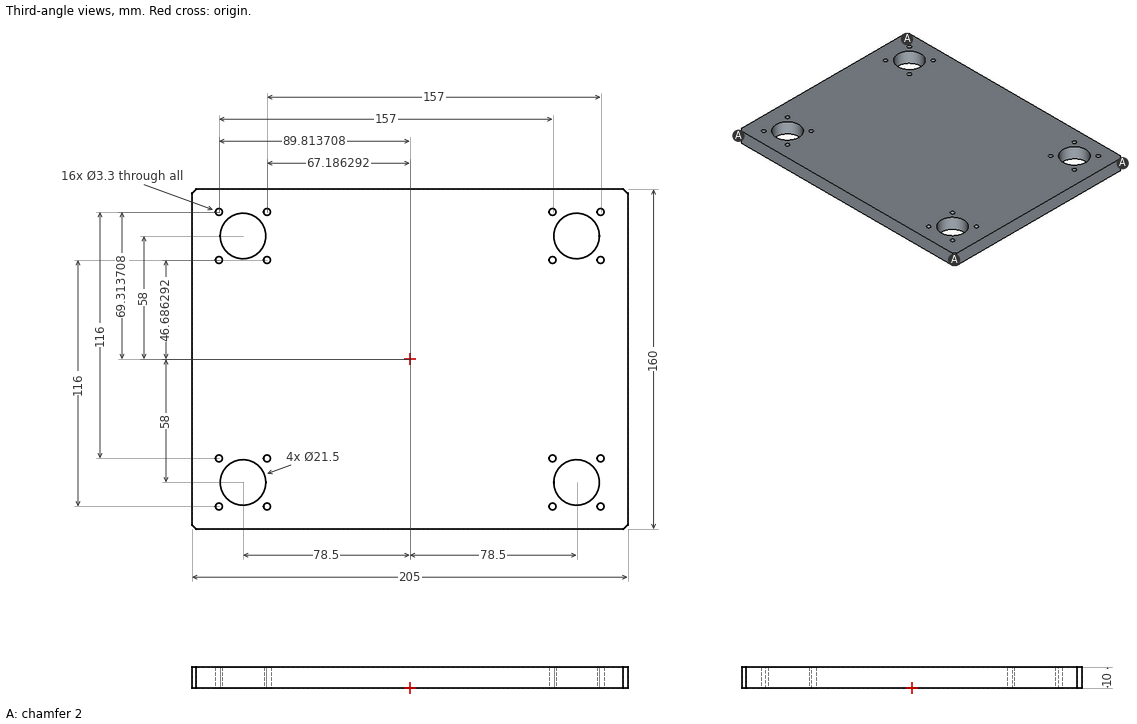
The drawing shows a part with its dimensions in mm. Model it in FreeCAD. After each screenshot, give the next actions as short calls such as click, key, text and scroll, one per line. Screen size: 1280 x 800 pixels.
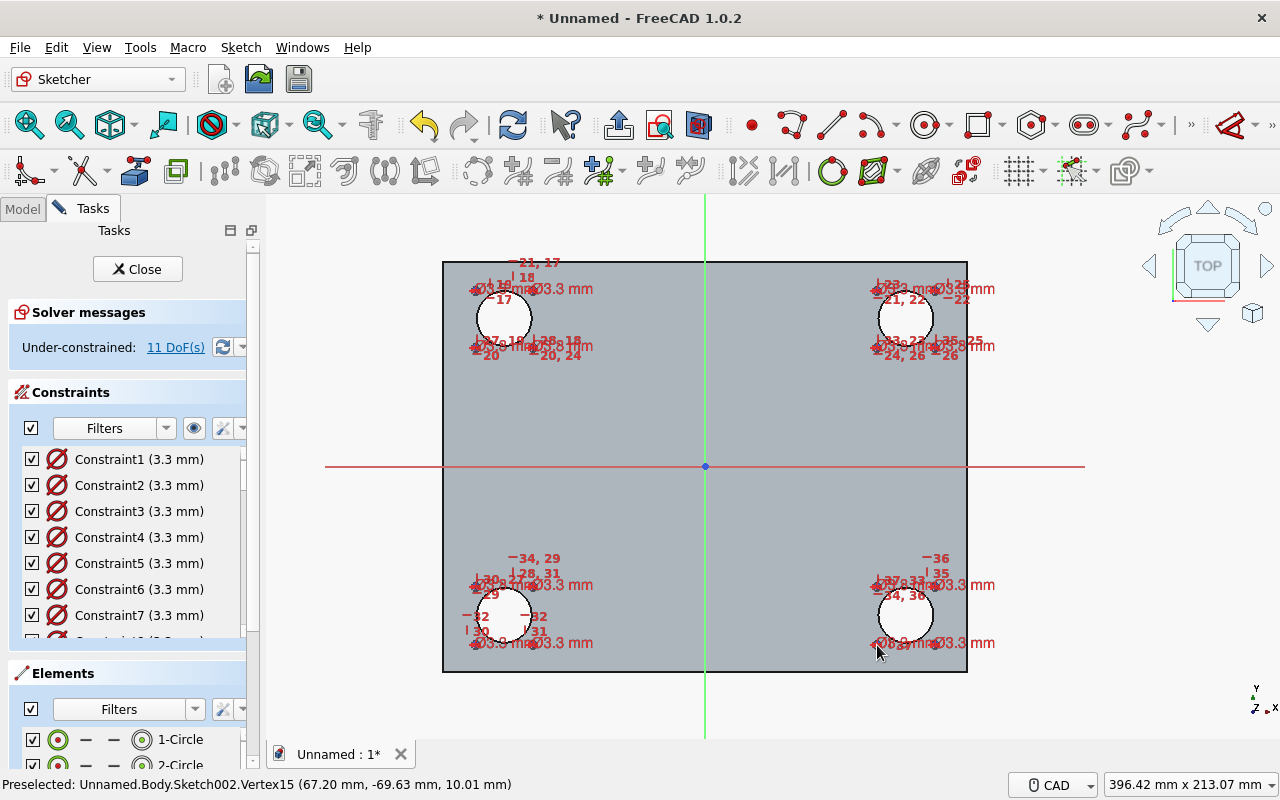
click(533, 645)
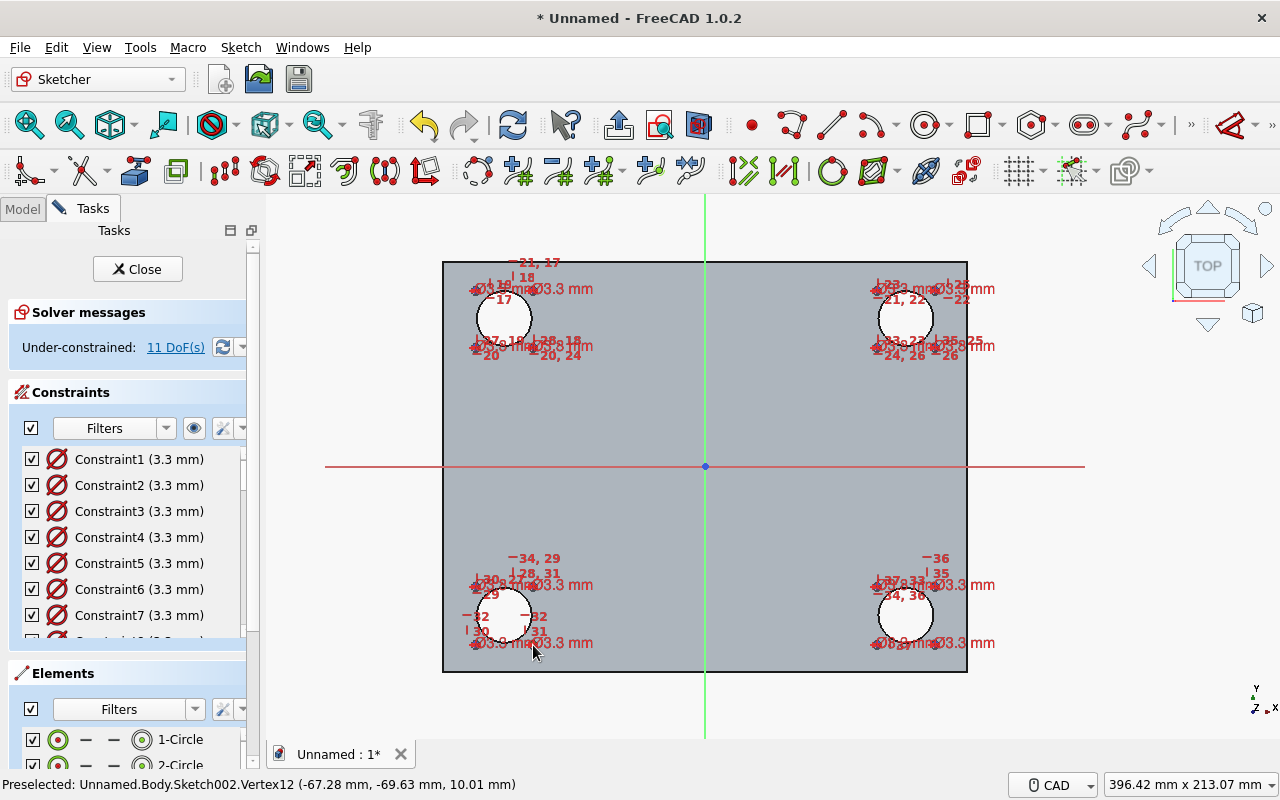
click(877, 645)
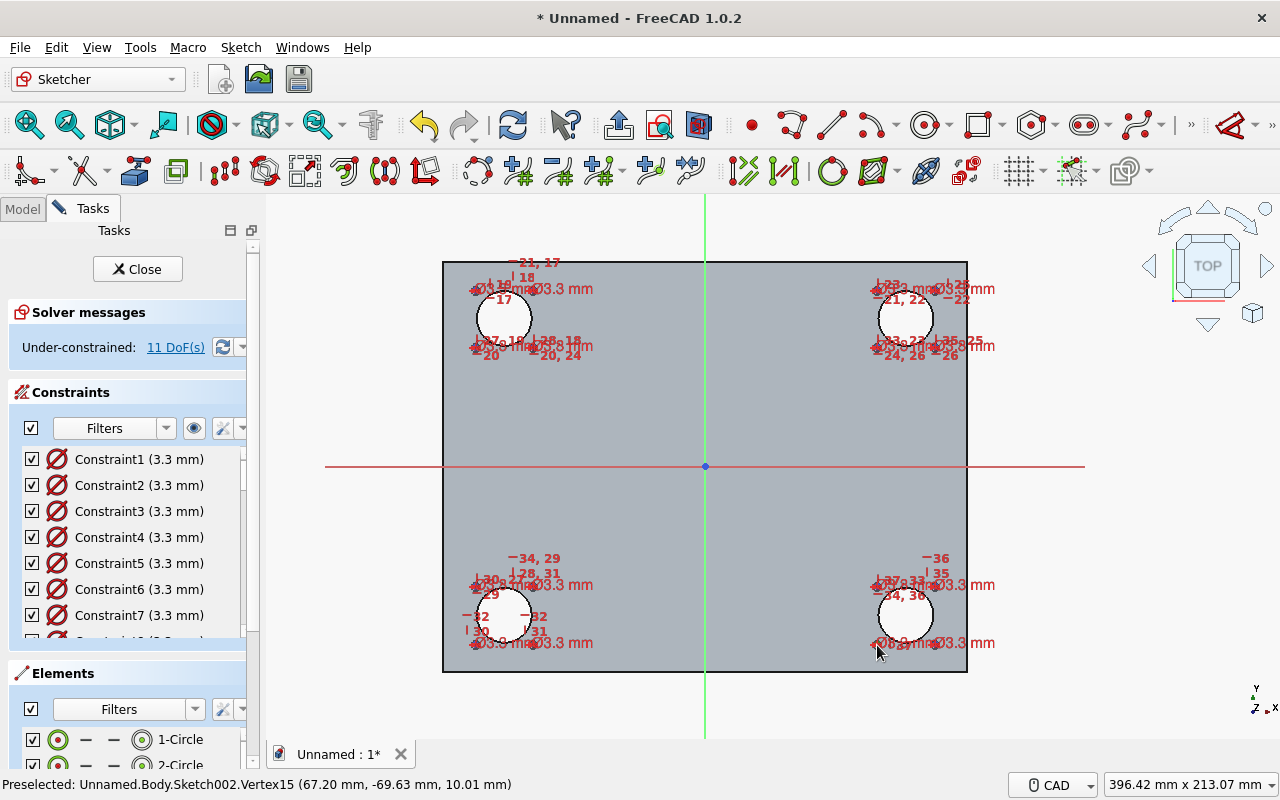
key(h)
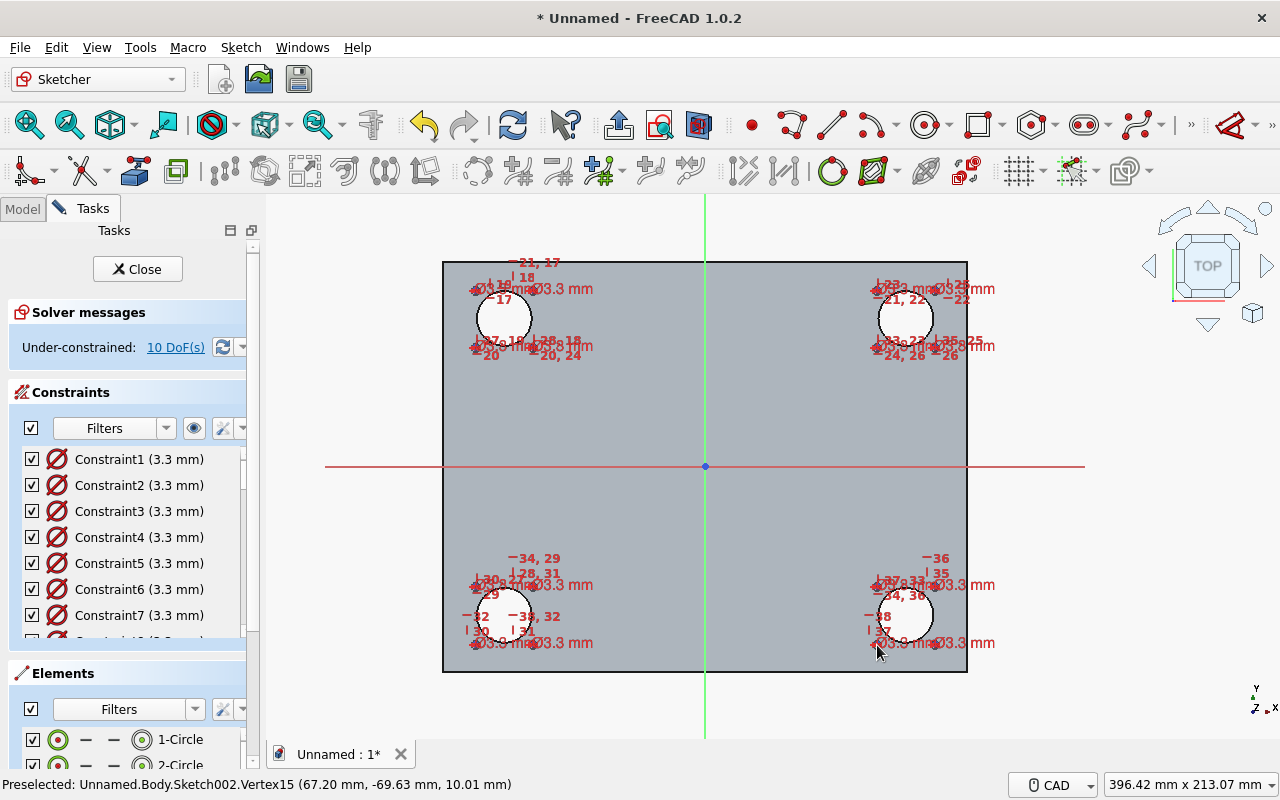
click(935, 587)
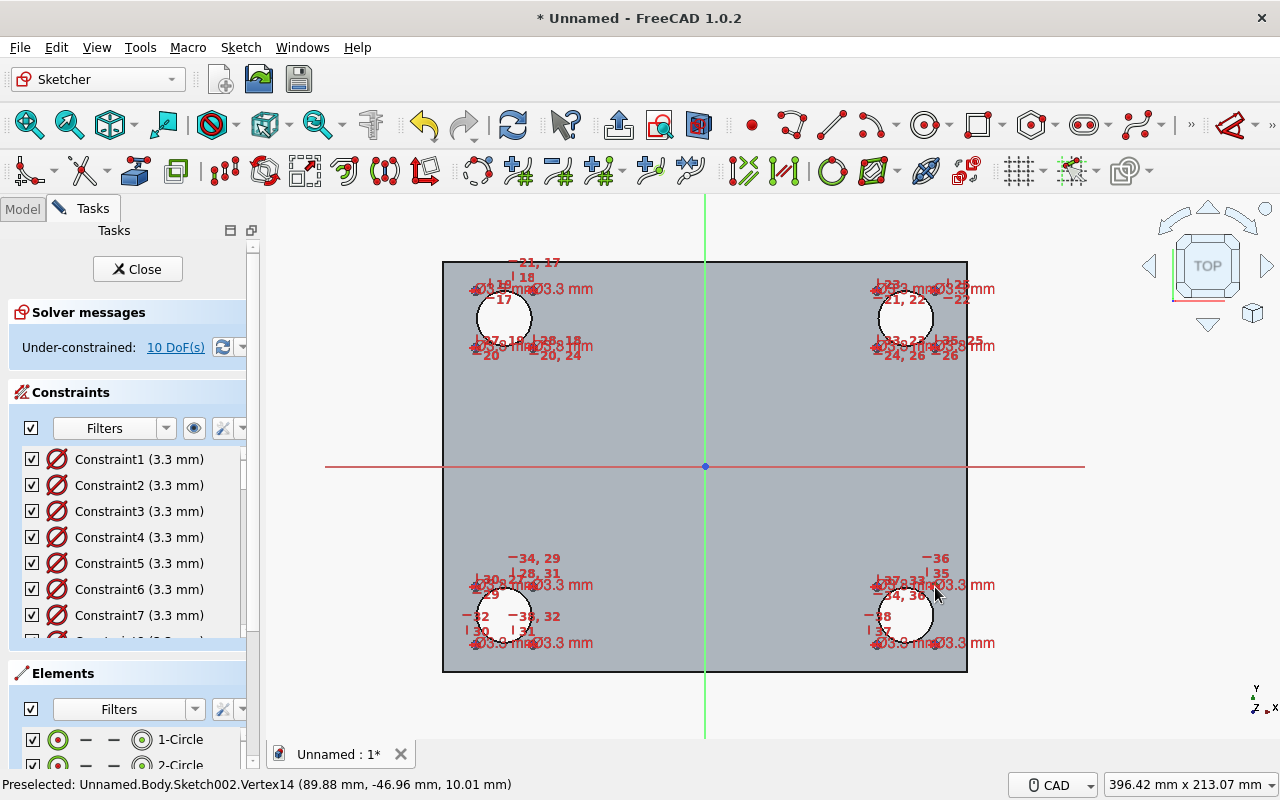
click(935, 645)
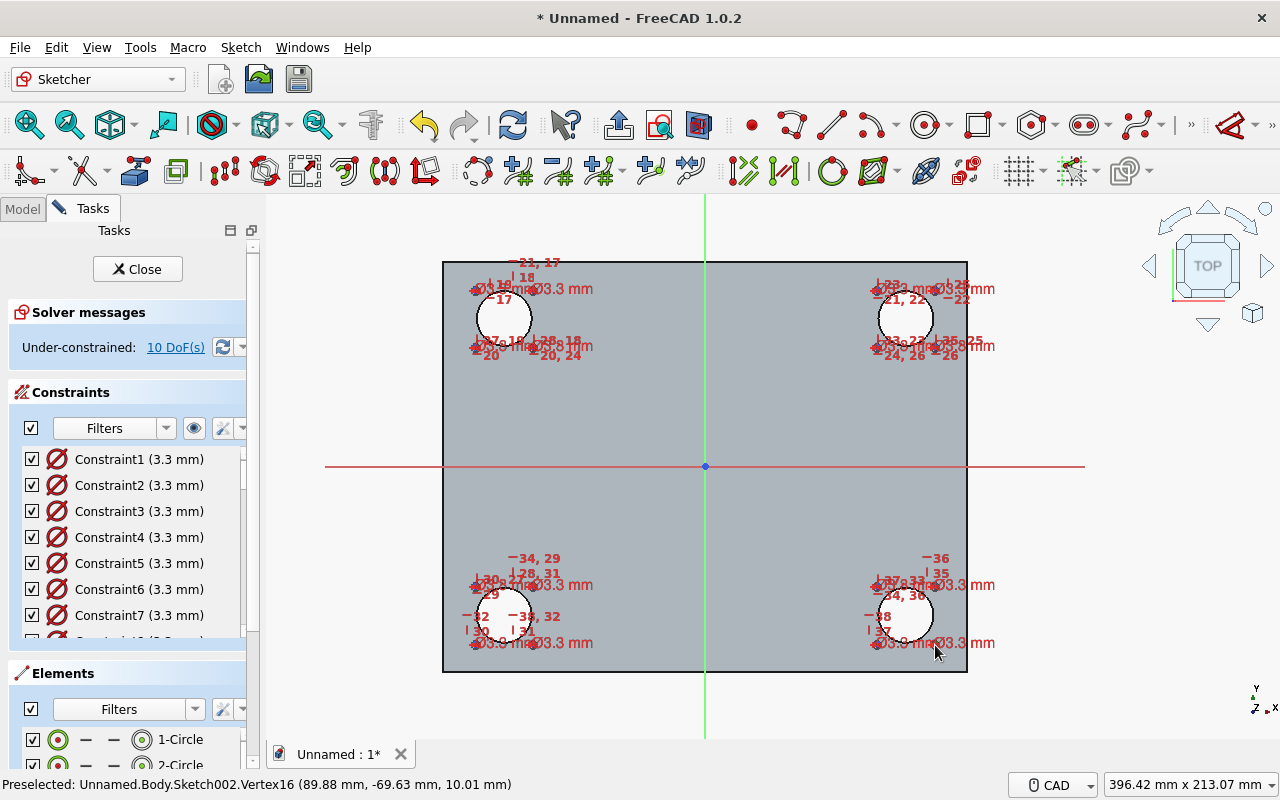
key(v)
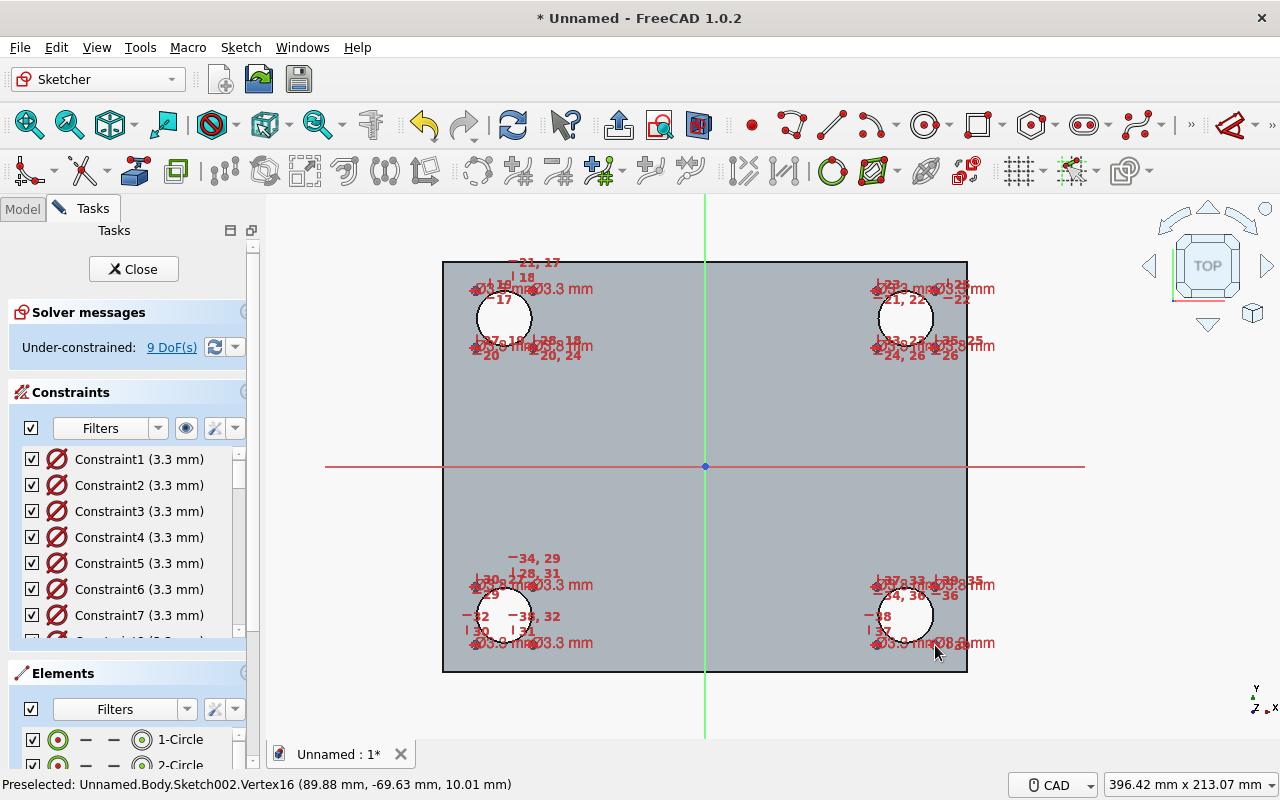
click(877, 645)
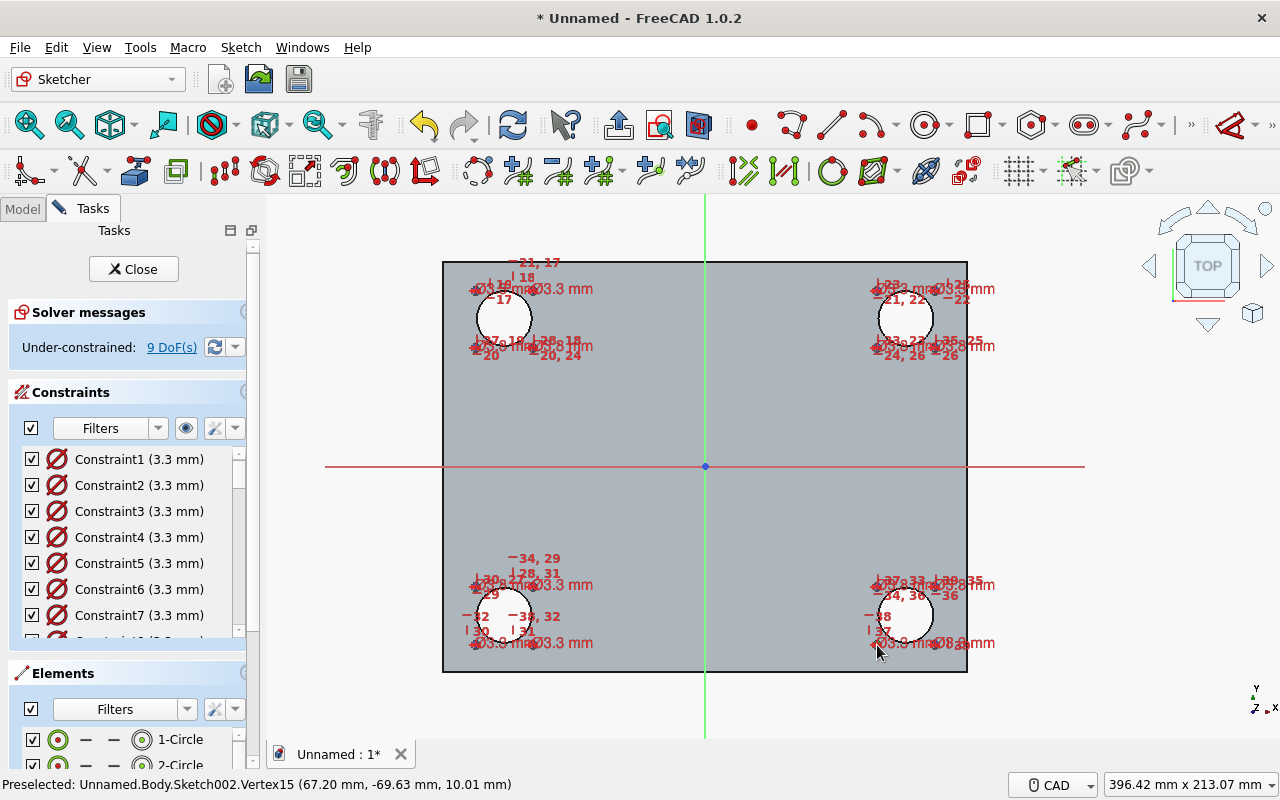
click(935, 645)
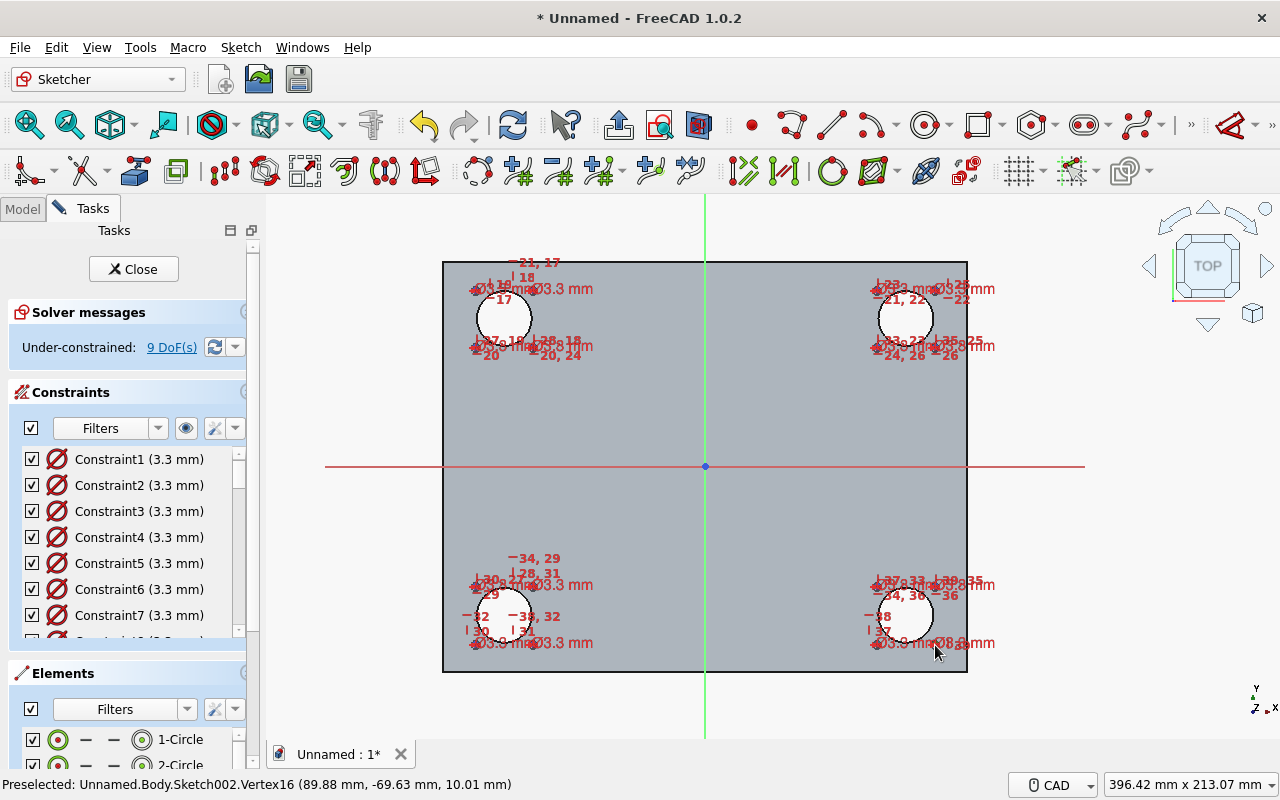
key(h)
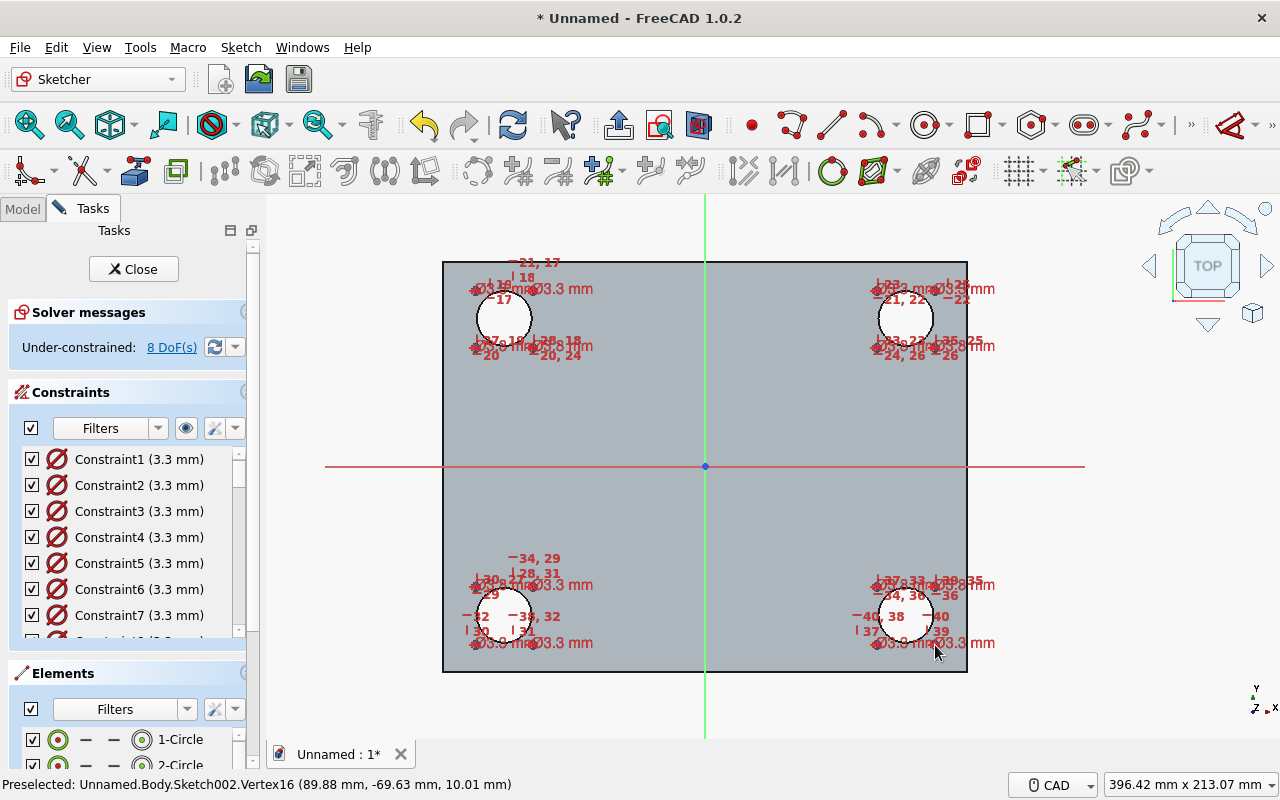
key(d)